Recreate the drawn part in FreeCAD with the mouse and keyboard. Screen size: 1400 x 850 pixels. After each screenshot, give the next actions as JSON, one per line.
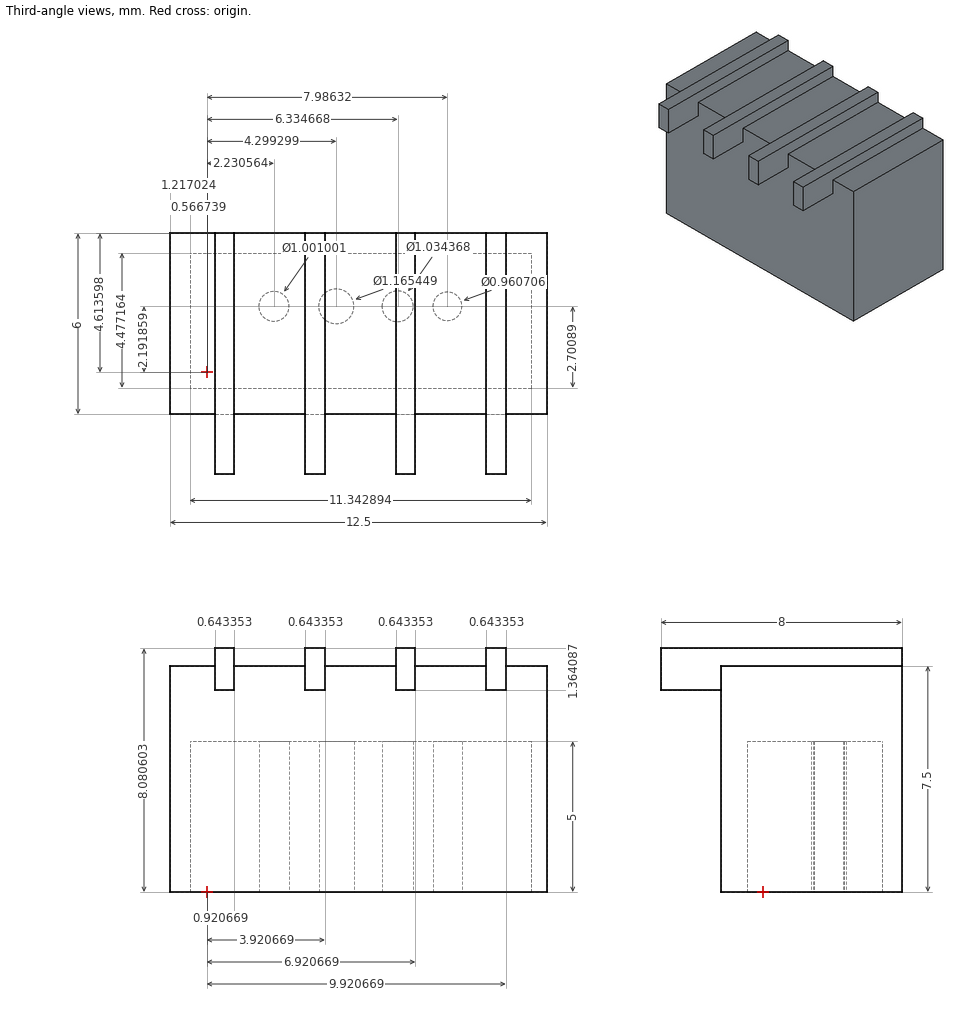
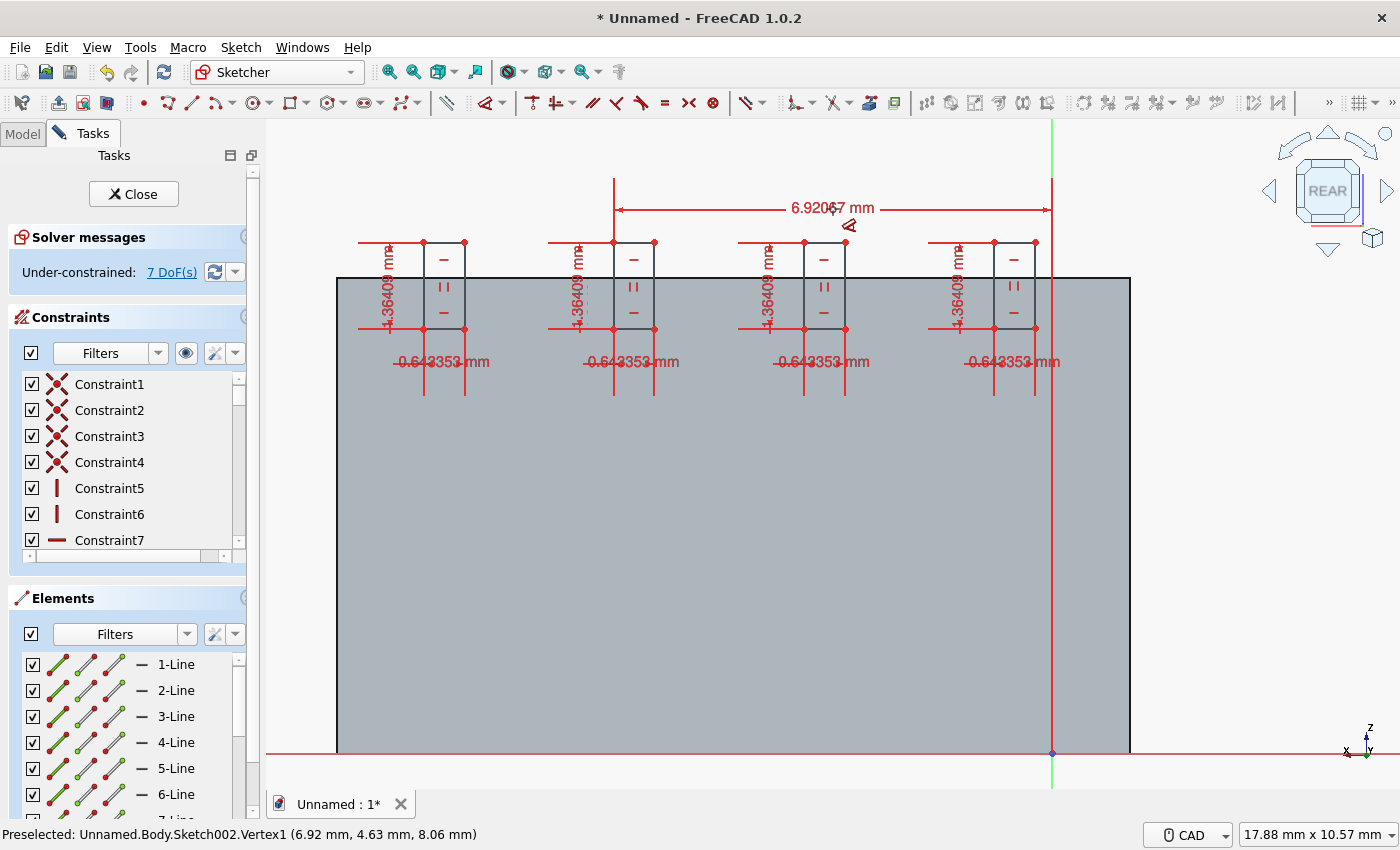
{"action": "left_click", "coordinate": [614, 243]}
{"action": "left_click", "coordinate": [1086, 498]}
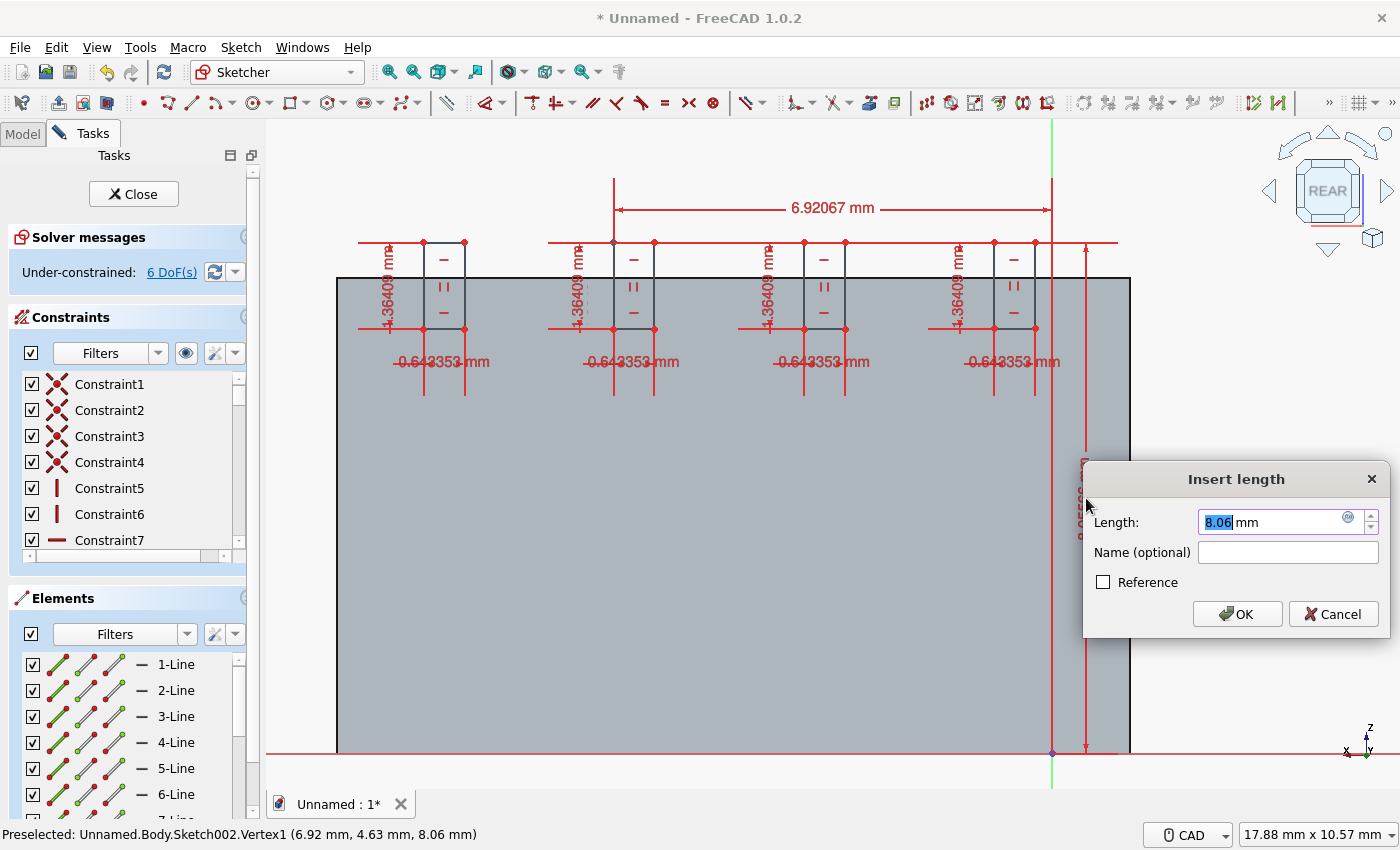
{"action": "type", "text": "8.080603"}
{"action": "key", "text": "Return"}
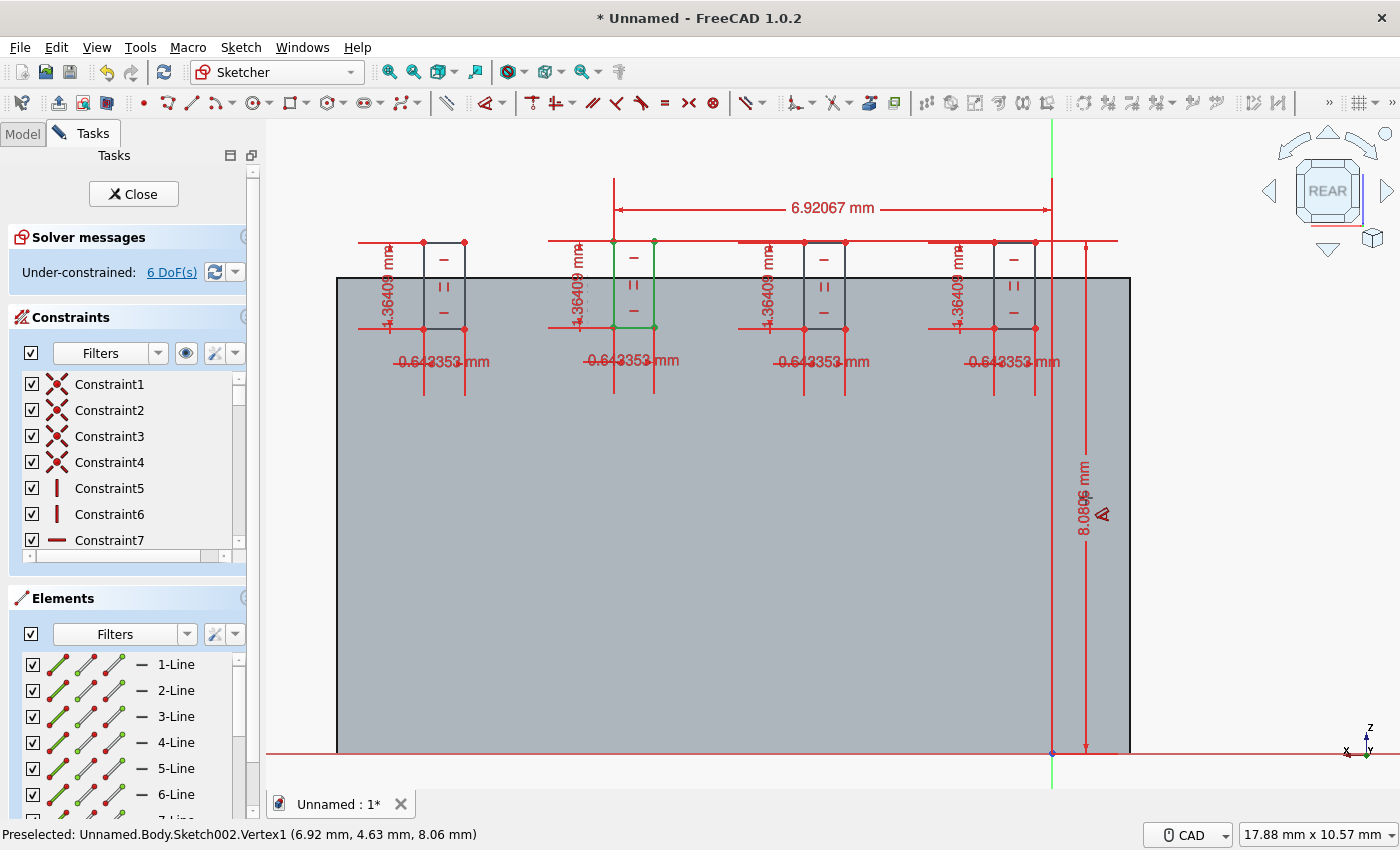
{"action": "left_click", "coordinate": [424, 243]}
{"action": "left_click", "coordinate": [738, 209]}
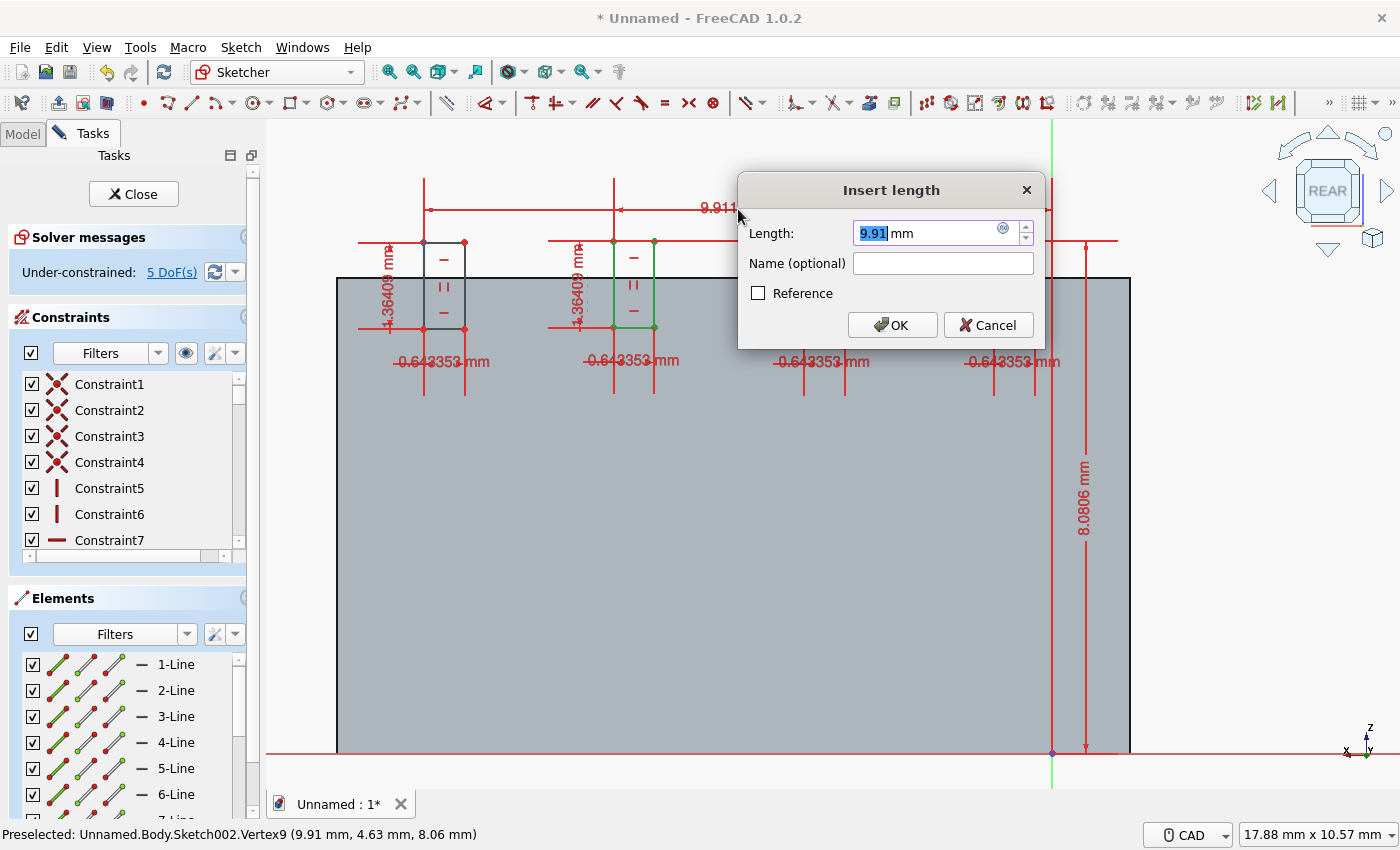
{"action": "type", "text": "9.920669"}
{"action": "key", "text": "Return"}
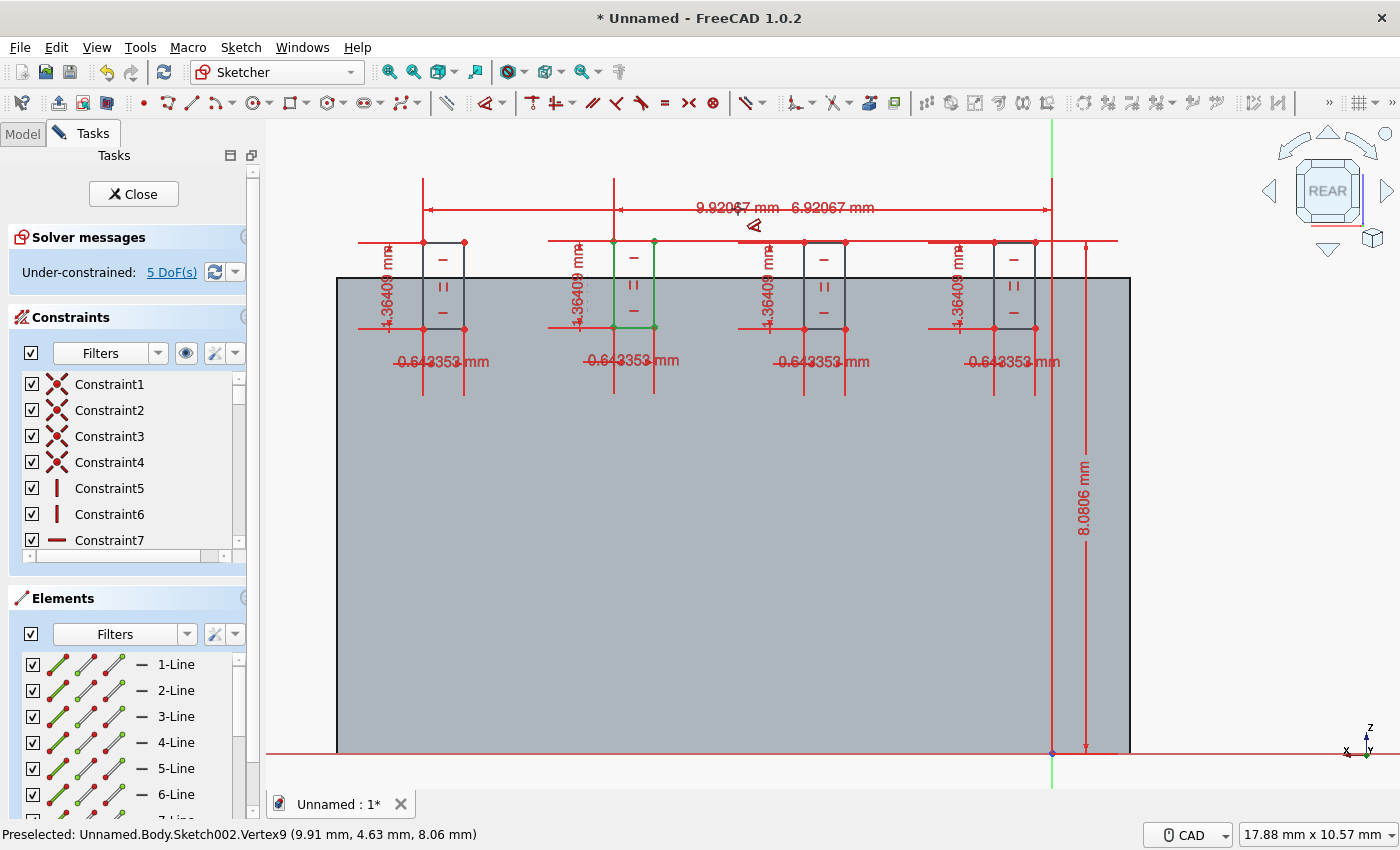
{"action": "left_click", "coordinate": [423, 243]}
{"action": "left_click", "coordinate": [389, 498]}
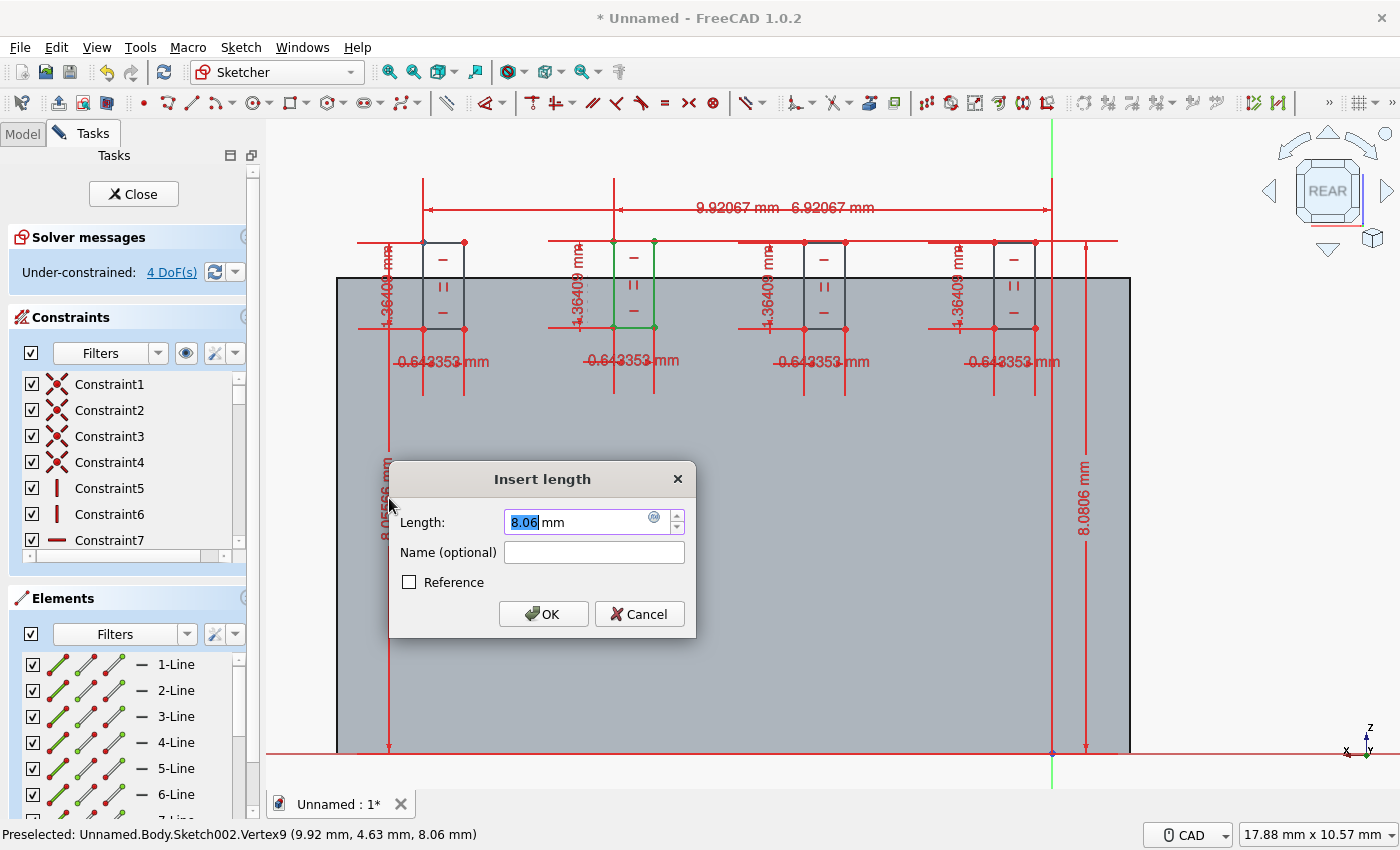
{"action": "type", "text": "8.080603"}
{"action": "key", "text": "Return"}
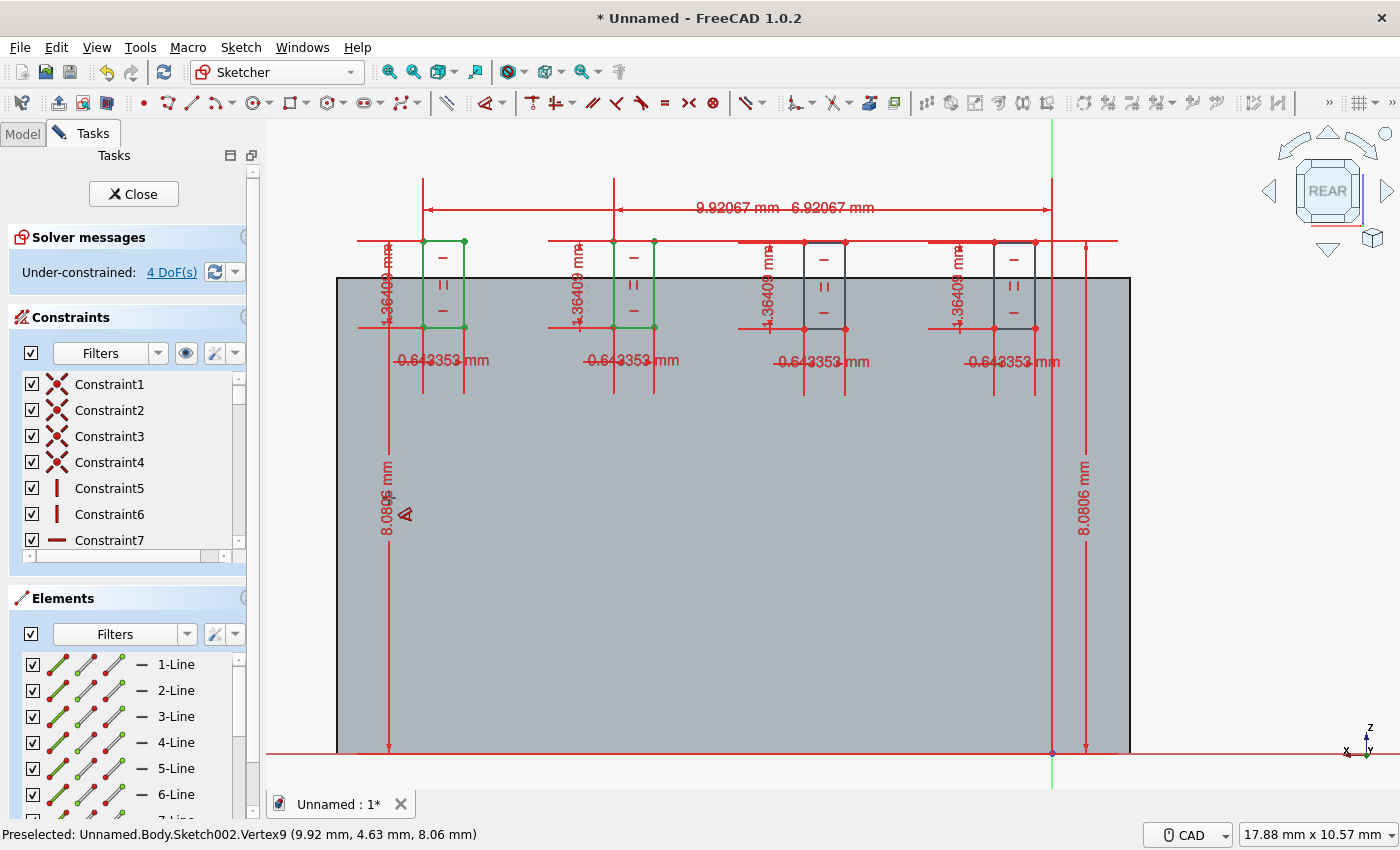
{"action": "left_click", "coordinate": [804, 243]}
{"action": "left_click", "coordinate": [928, 209]}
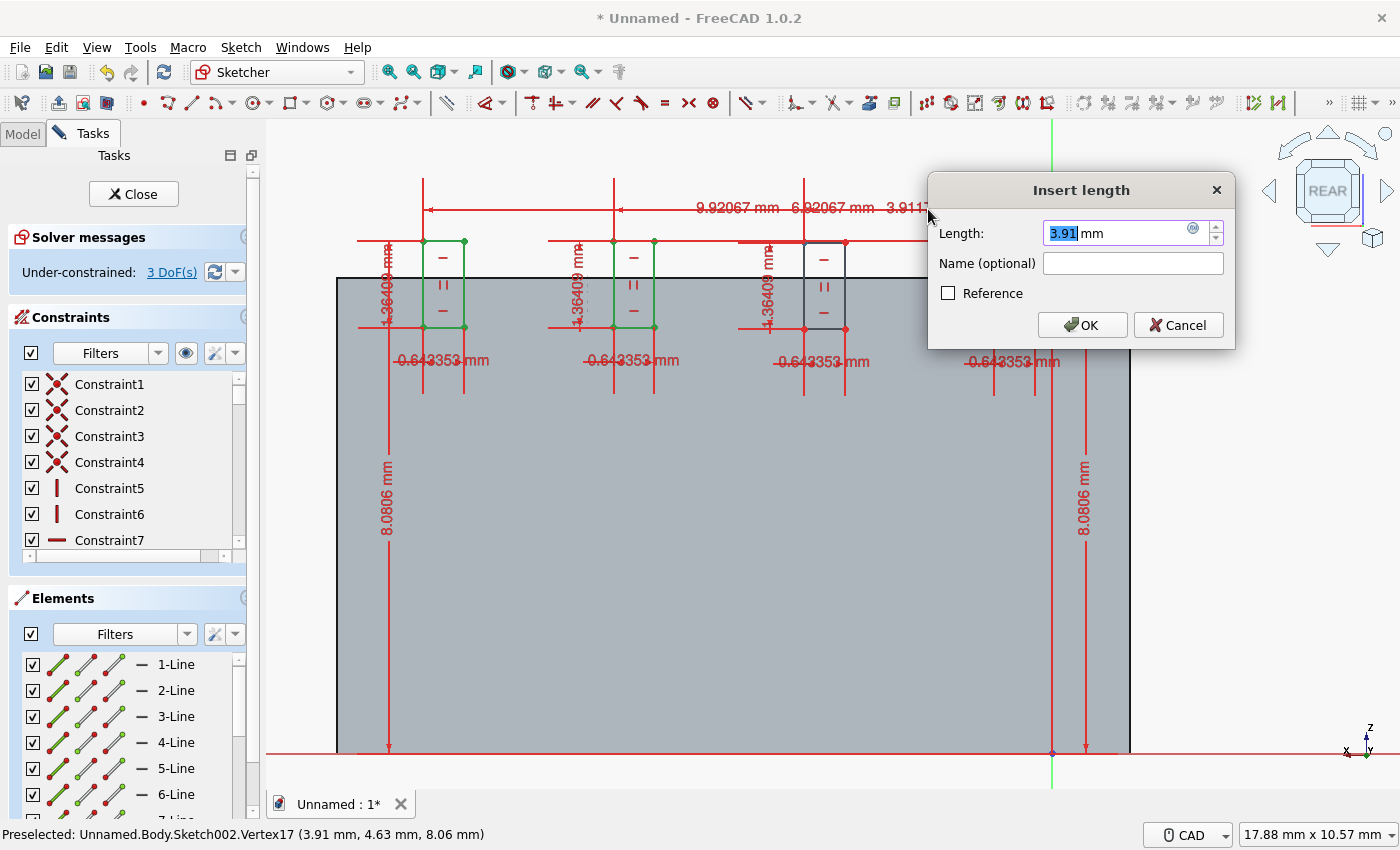
{"action": "type", "text": "3.920669"}
{"action": "key", "text": "Return"}